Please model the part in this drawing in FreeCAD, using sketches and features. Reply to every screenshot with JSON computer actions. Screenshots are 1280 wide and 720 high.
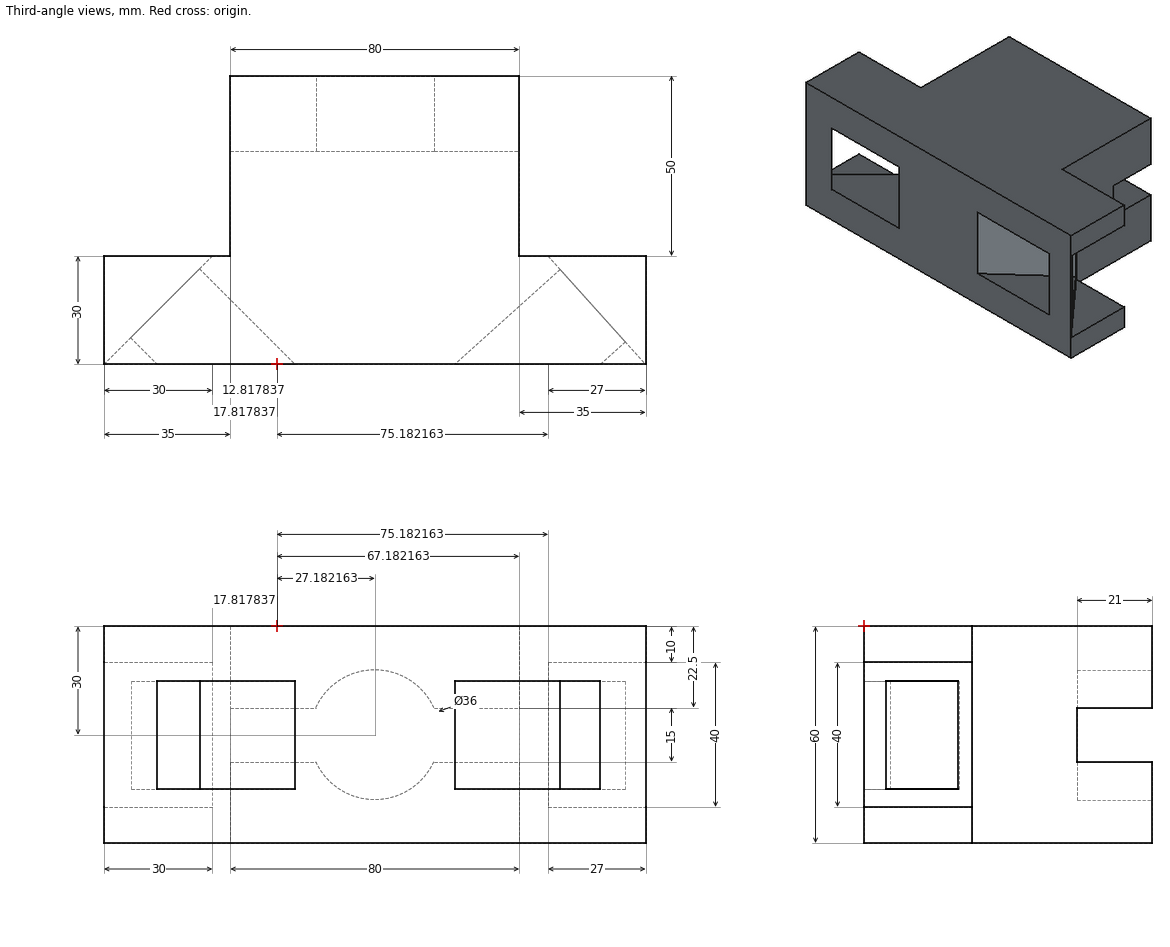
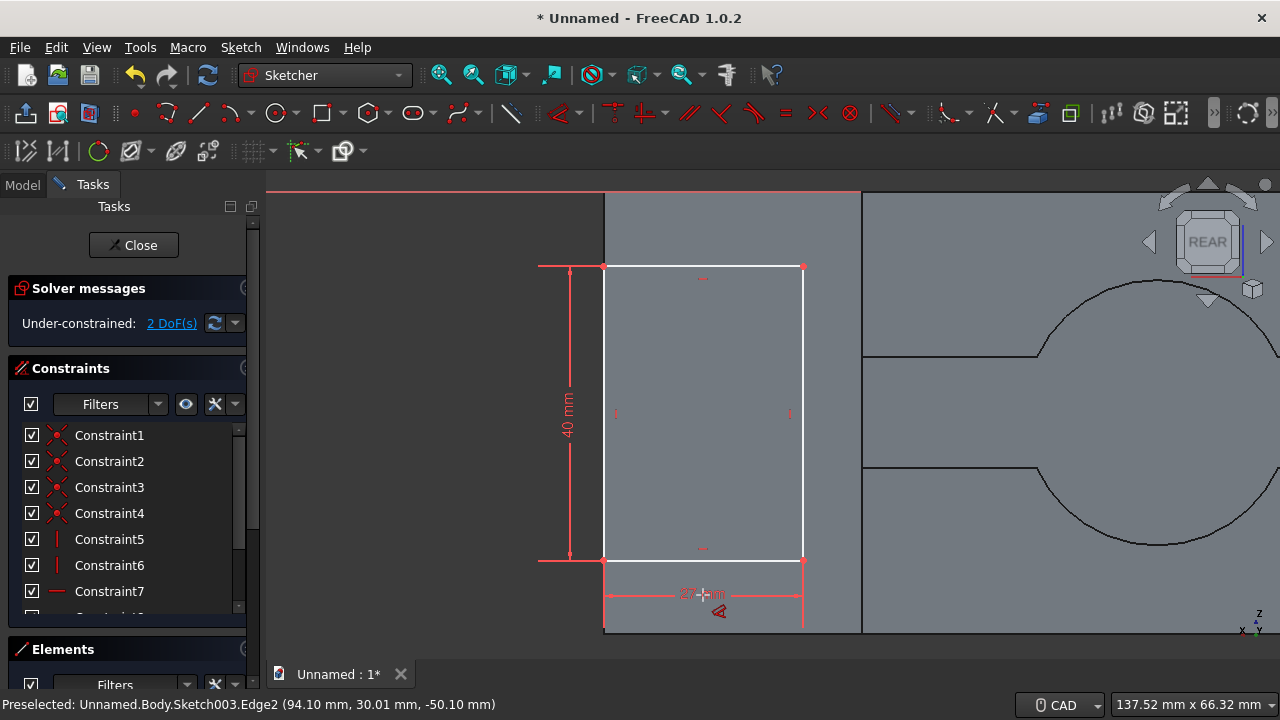
{"action": "left_click", "coordinate": [604, 266]}
{"action": "left_click", "coordinate": [570, 232]}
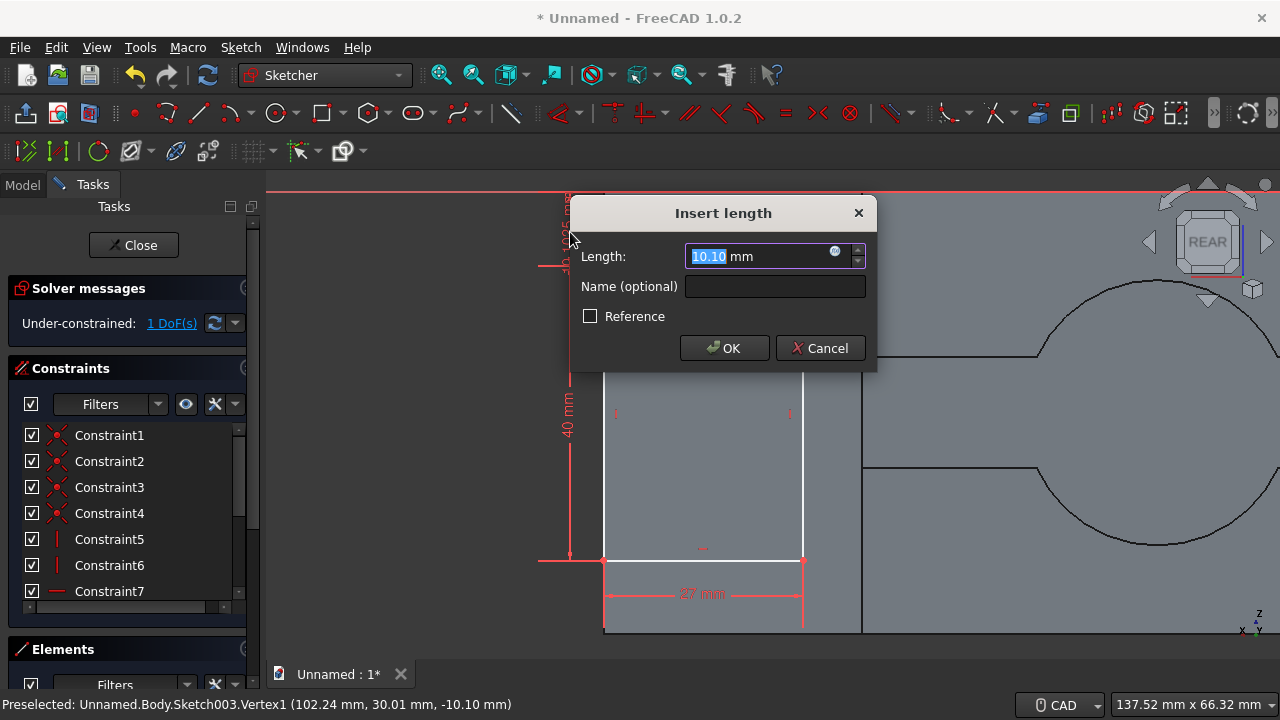
{"action": "type", "text": "10"}
{"action": "key", "text": "Return"}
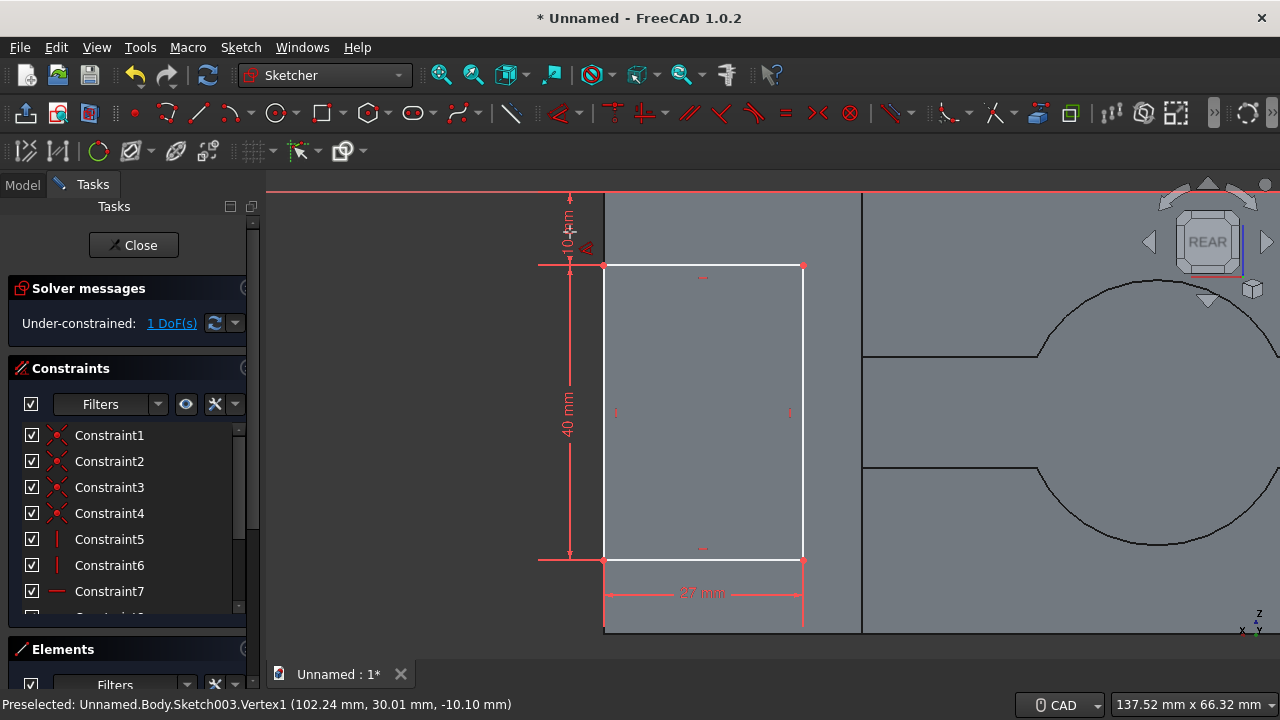
{"action": "left_click", "coordinate": [803, 560]}
{"action": "left_click", "coordinate": [959, 594]}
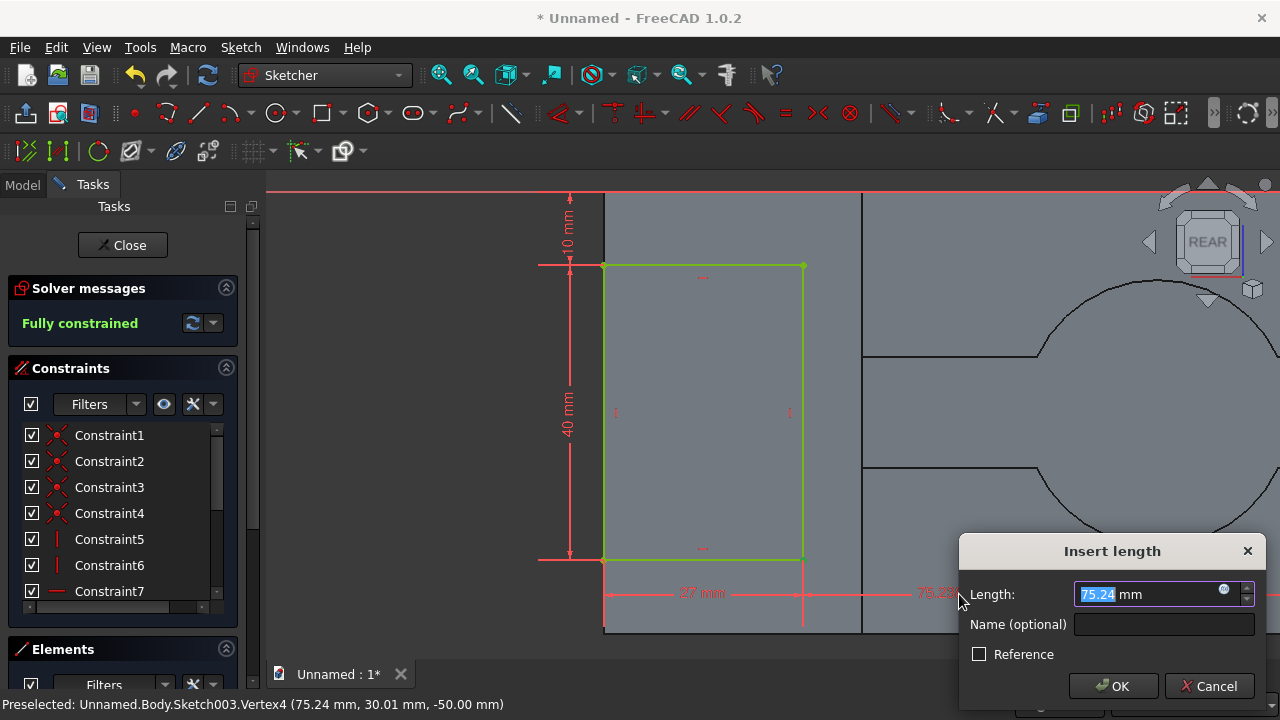
{"action": "type", "text": "75.182163"}
{"action": "key", "text": "Return"}
{"action": "key", "text": "Escape"}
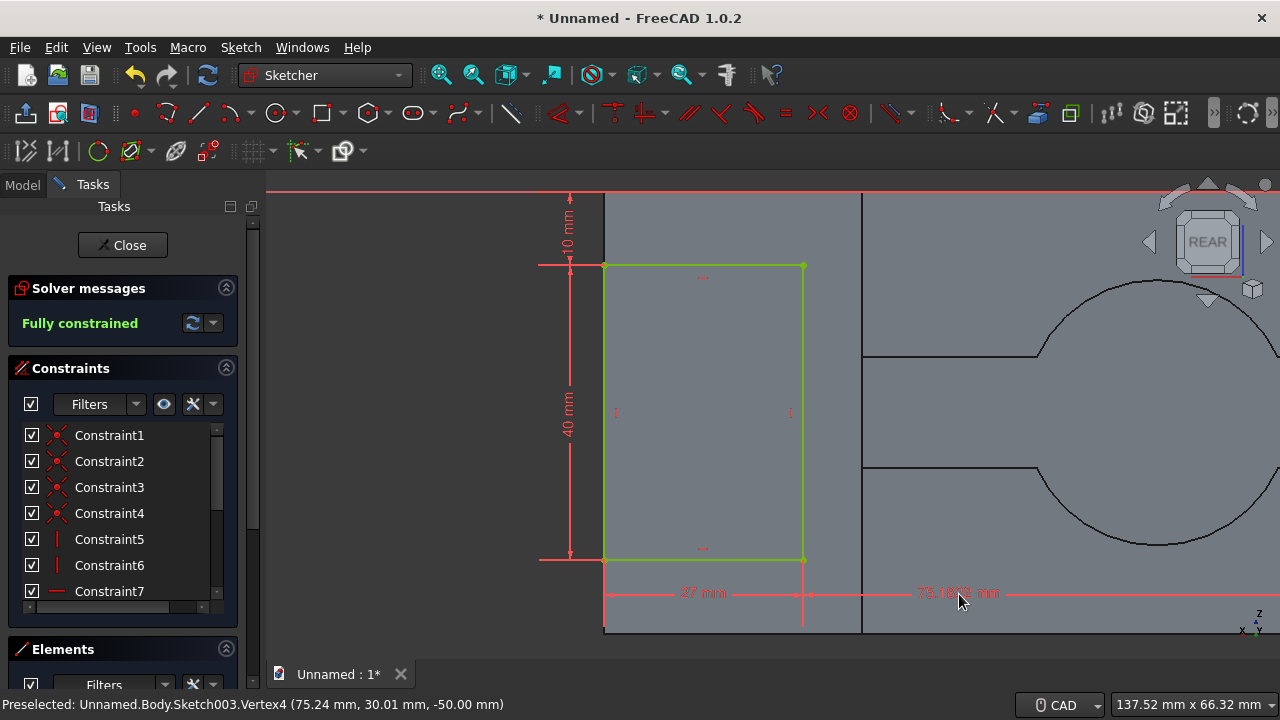
{"action": "left_click", "coordinate": [123, 245]}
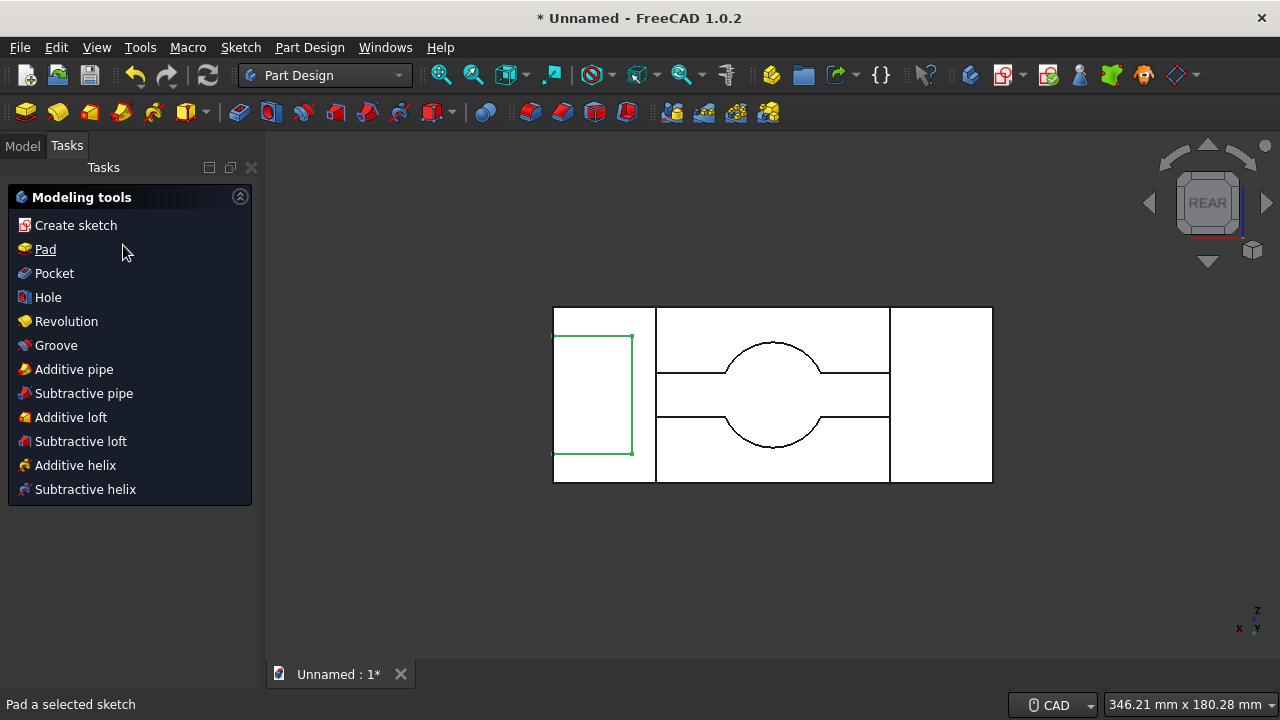
{"action": "left_click", "coordinate": [240, 112]}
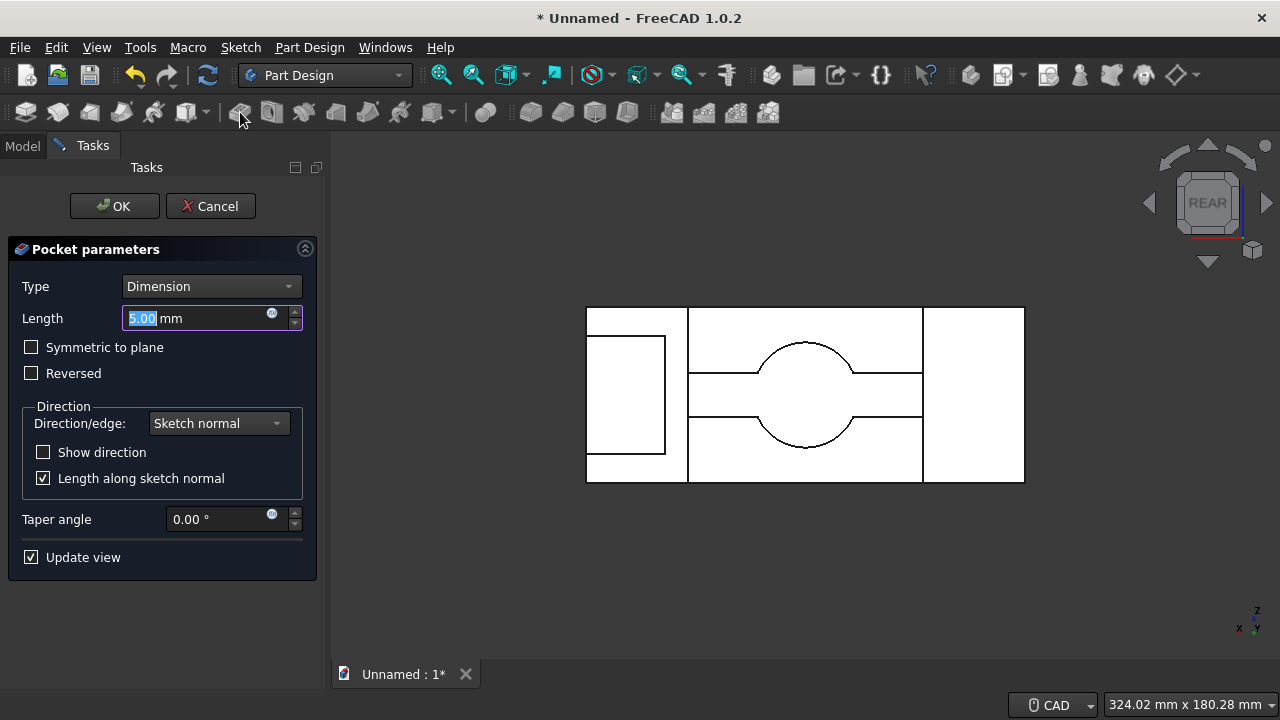
{"action": "type", "text": "40"}
{"action": "key", "text": "Tab"}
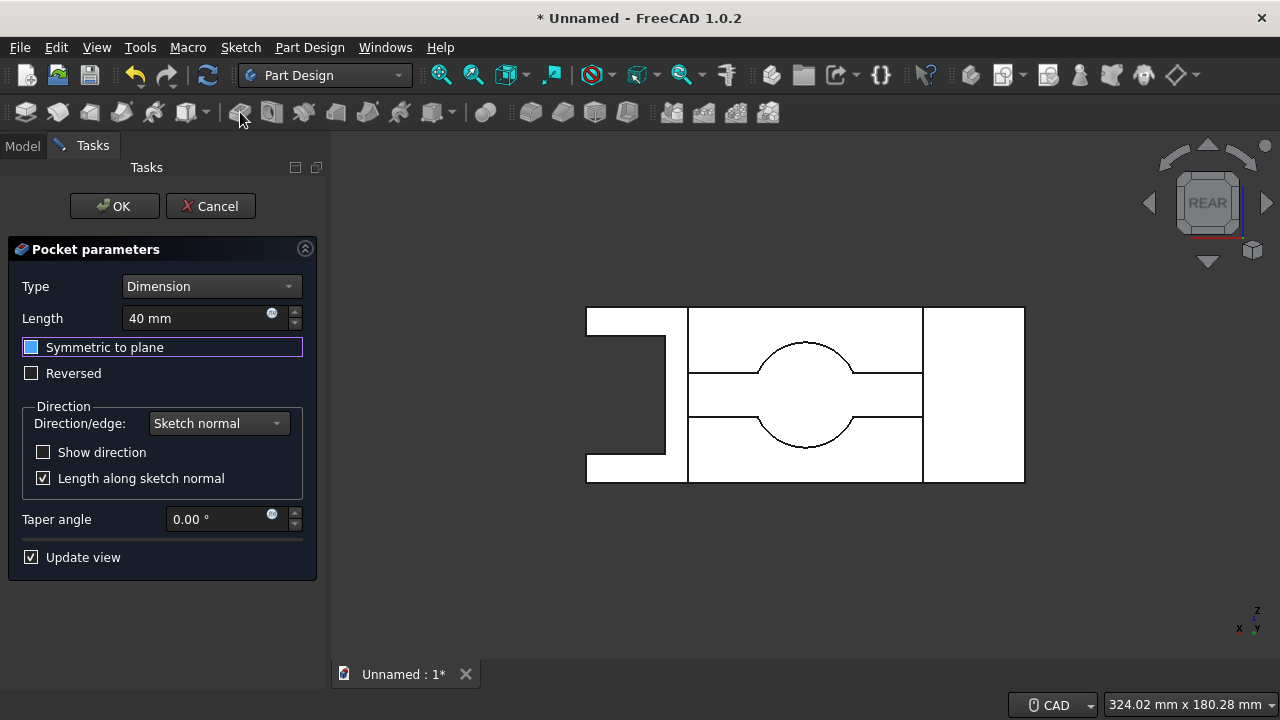
{"action": "left_click", "coordinate": [115, 206]}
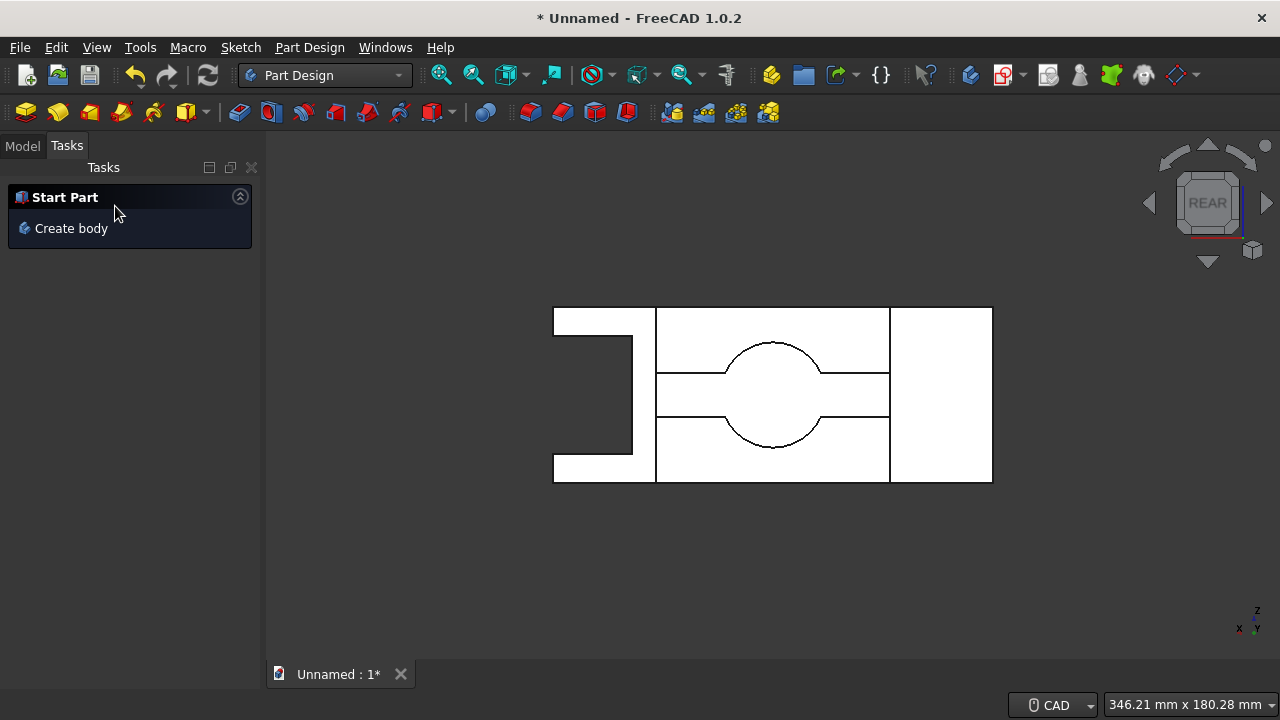
{"action": "left_click", "coordinate": [442, 76]}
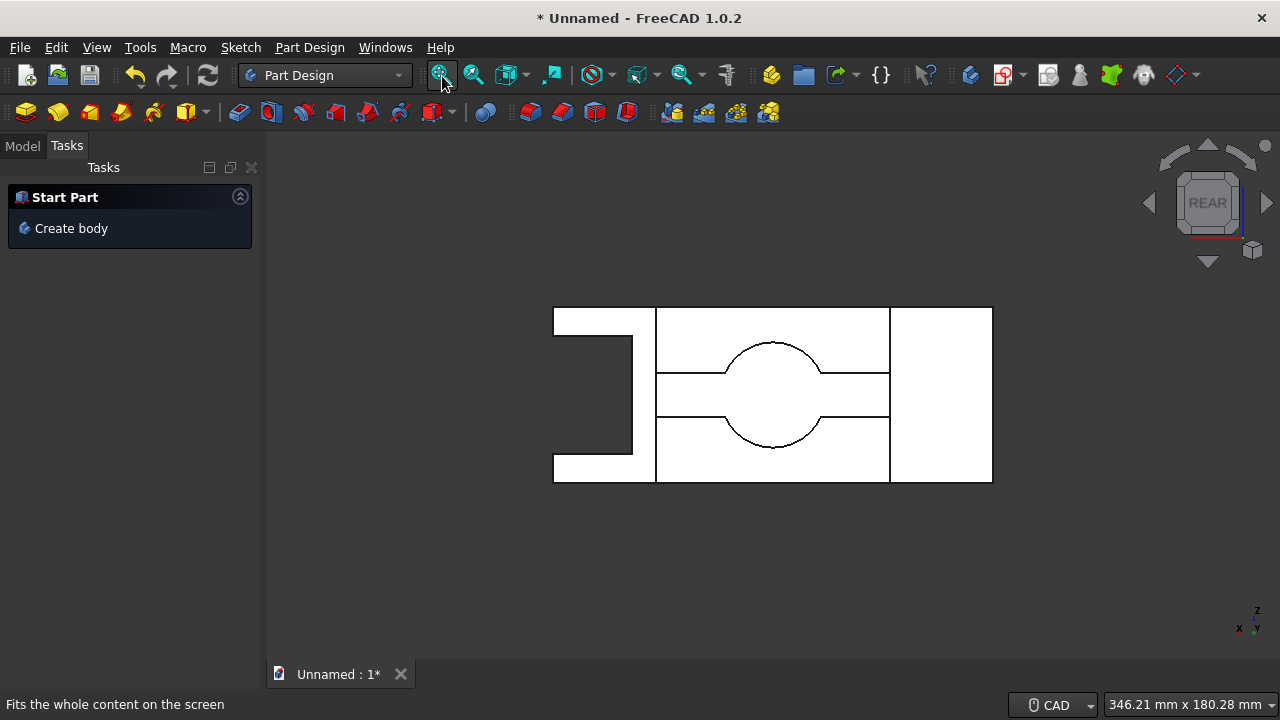
{"action": "left_click", "coordinate": [23, 145]}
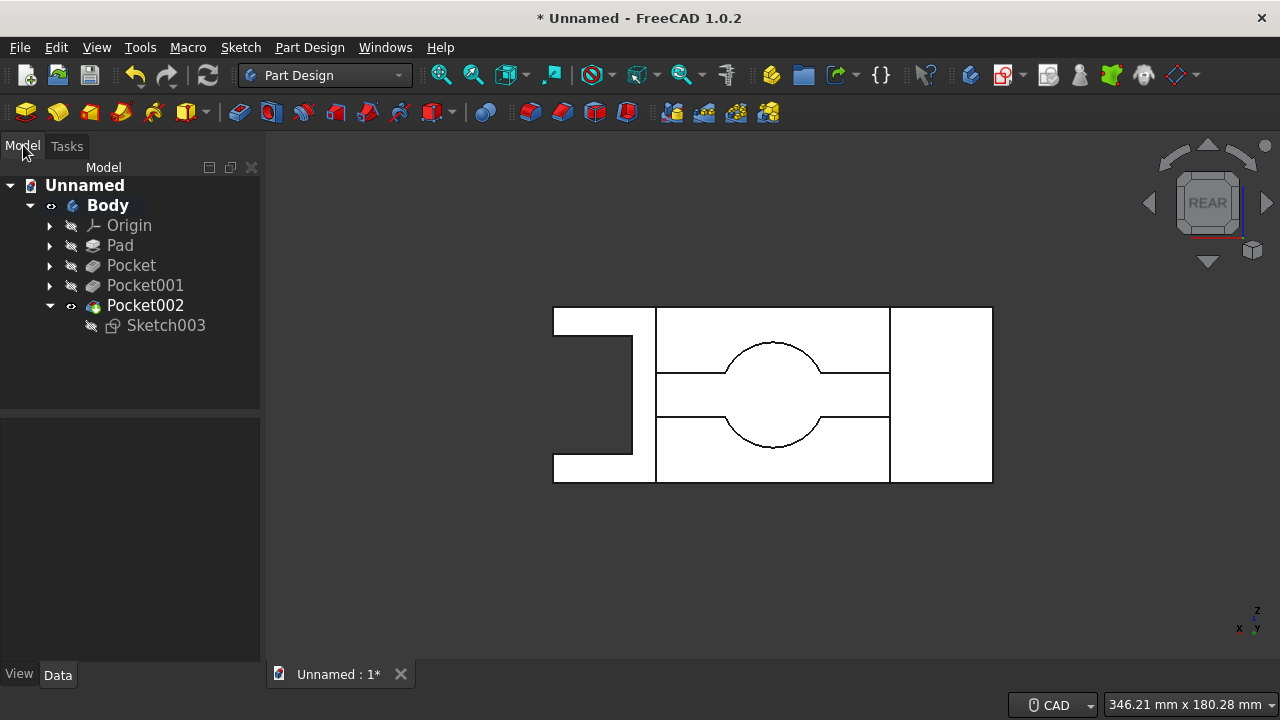
{"action": "left_click", "coordinate": [50, 226]}